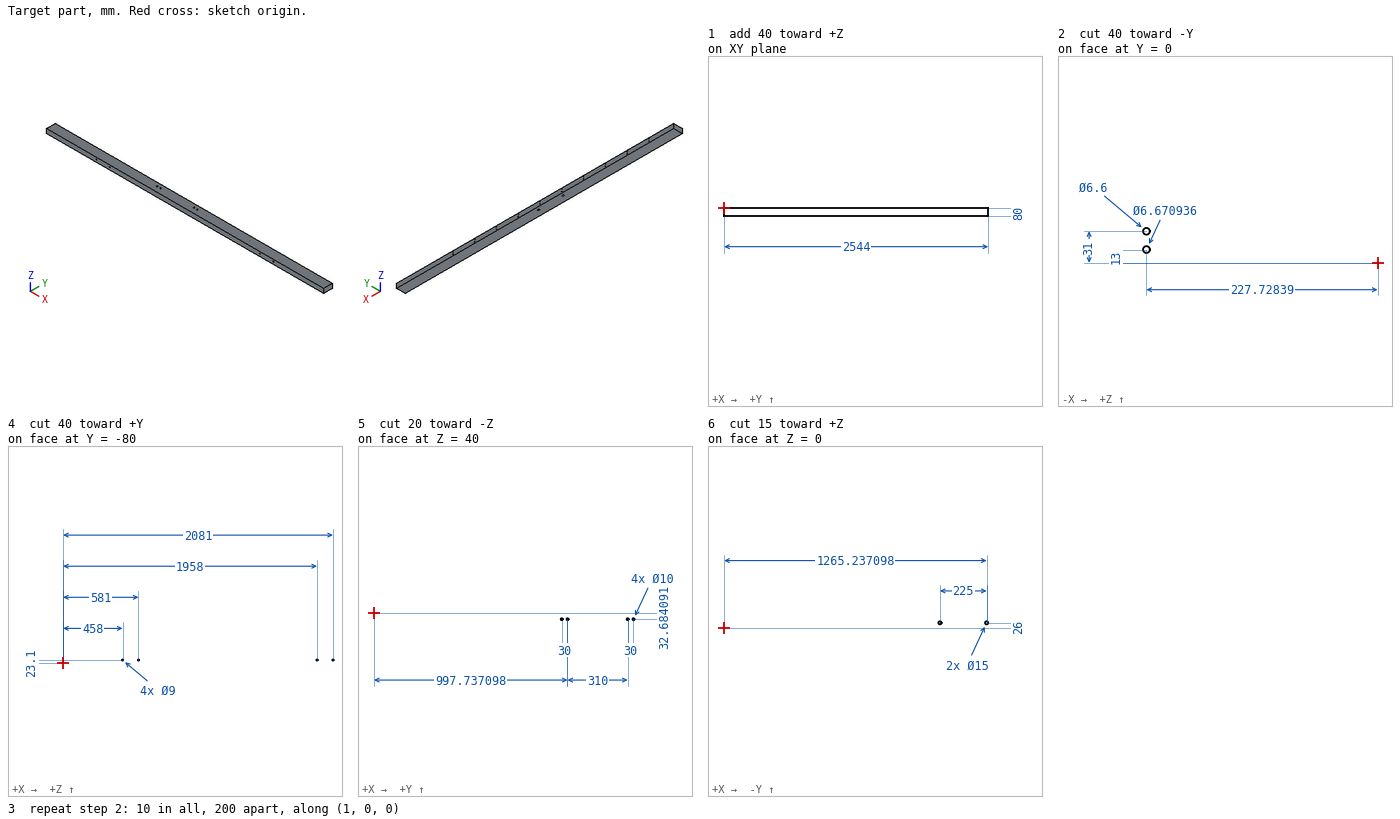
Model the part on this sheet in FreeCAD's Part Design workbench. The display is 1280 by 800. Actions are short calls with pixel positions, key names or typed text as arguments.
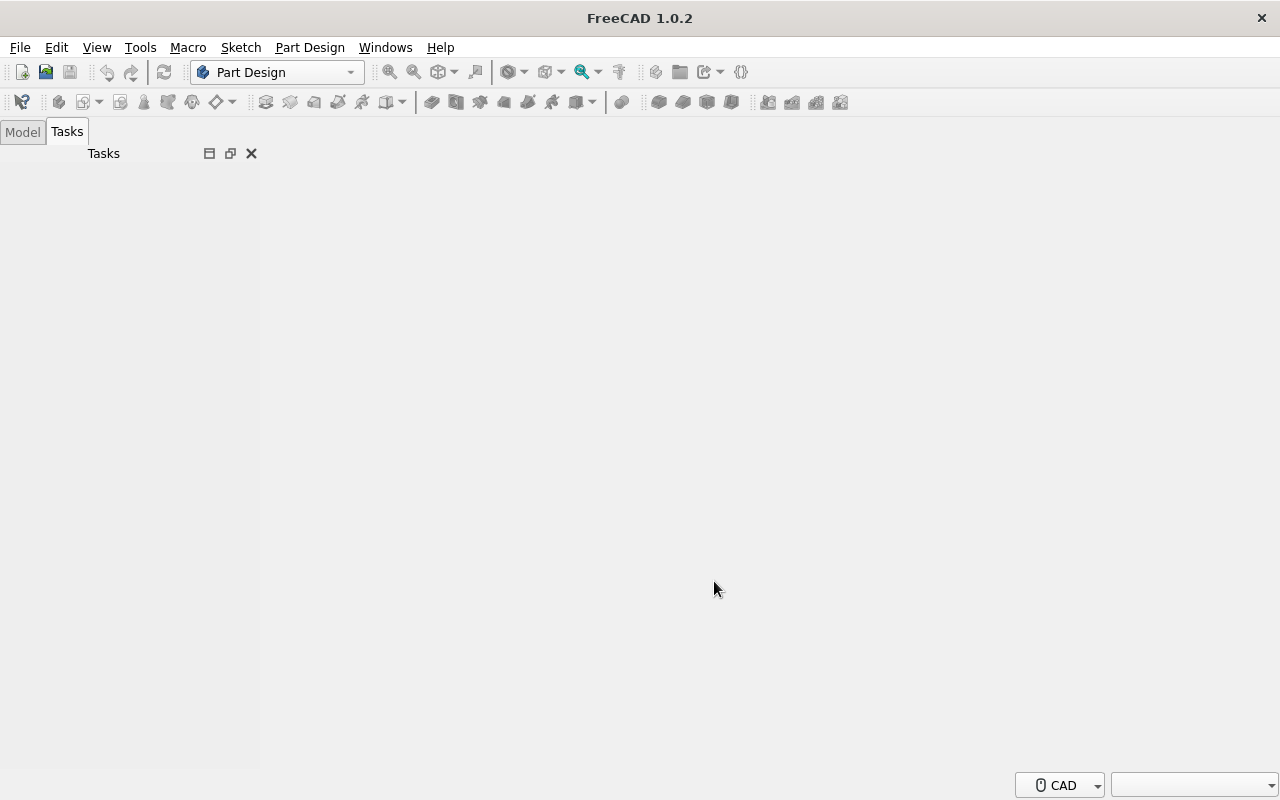
key(ctrl+n)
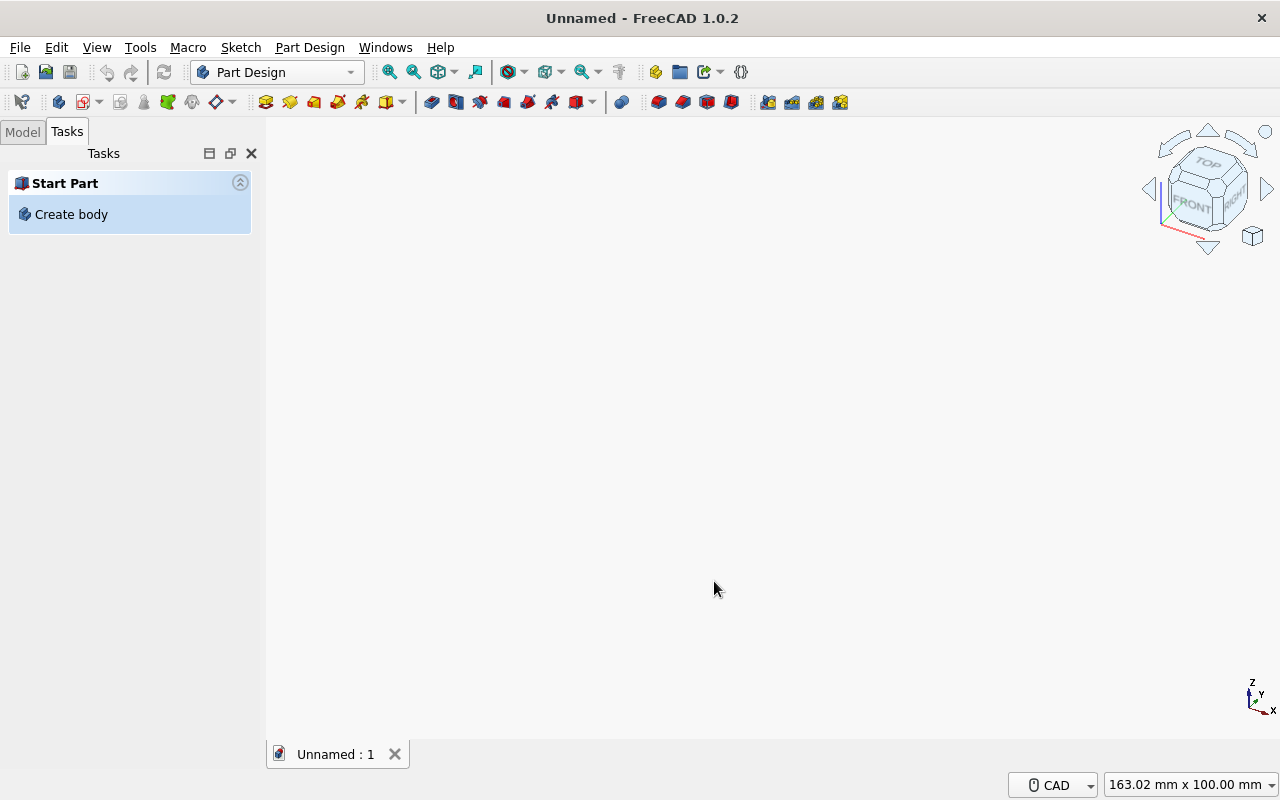
click(84, 102)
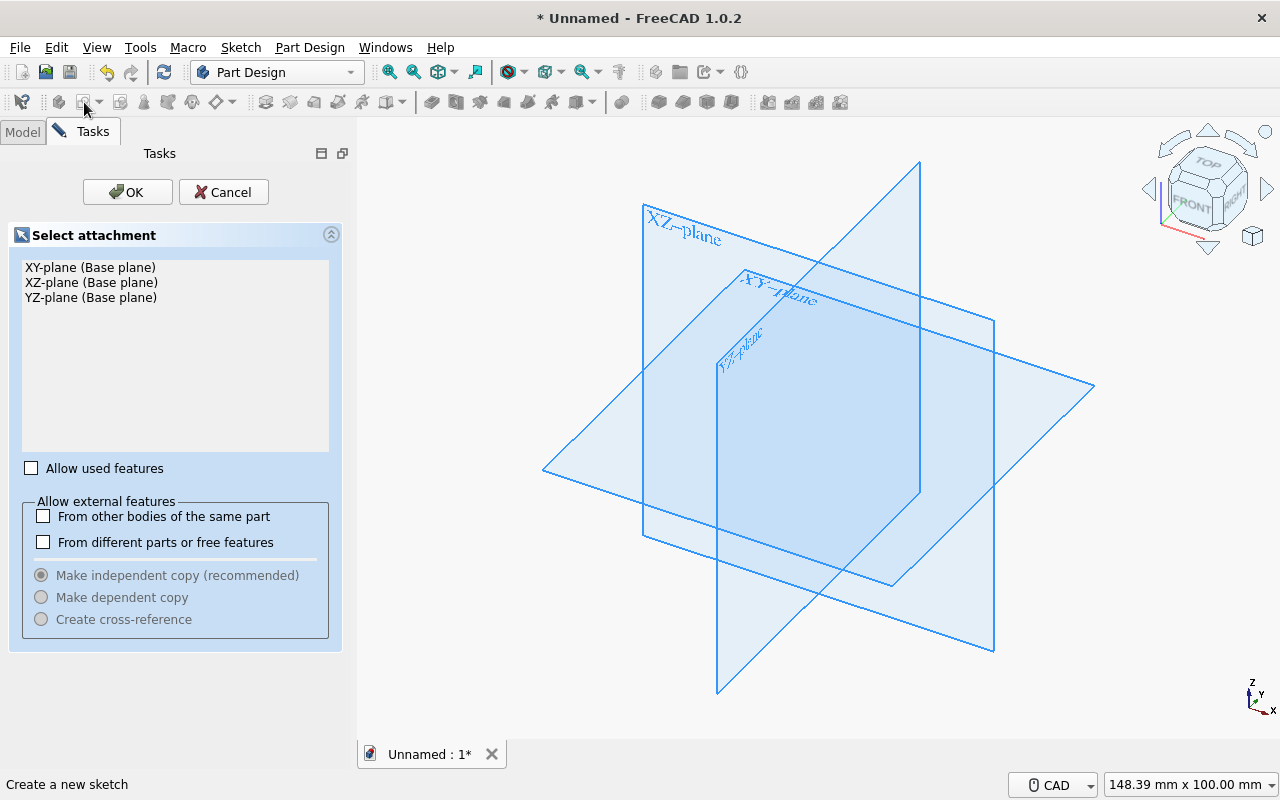
click(82, 268)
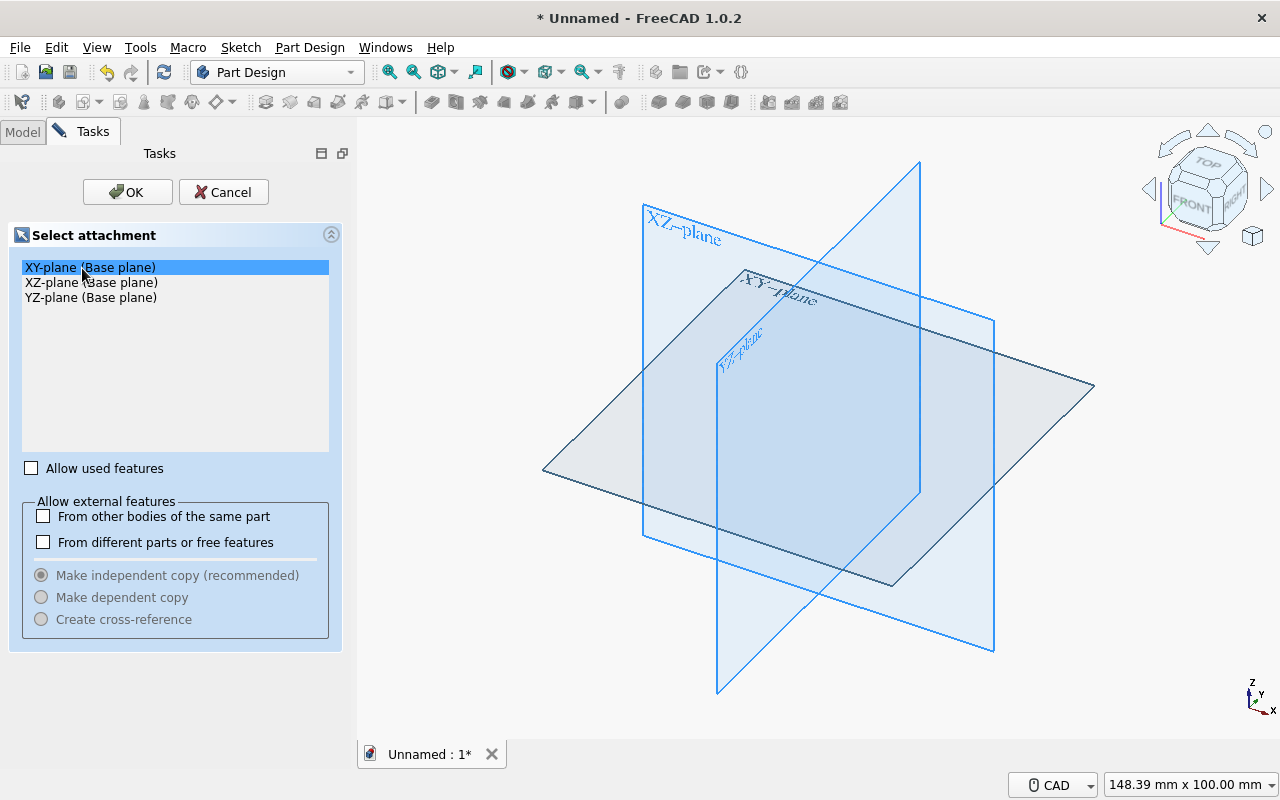
click(128, 192)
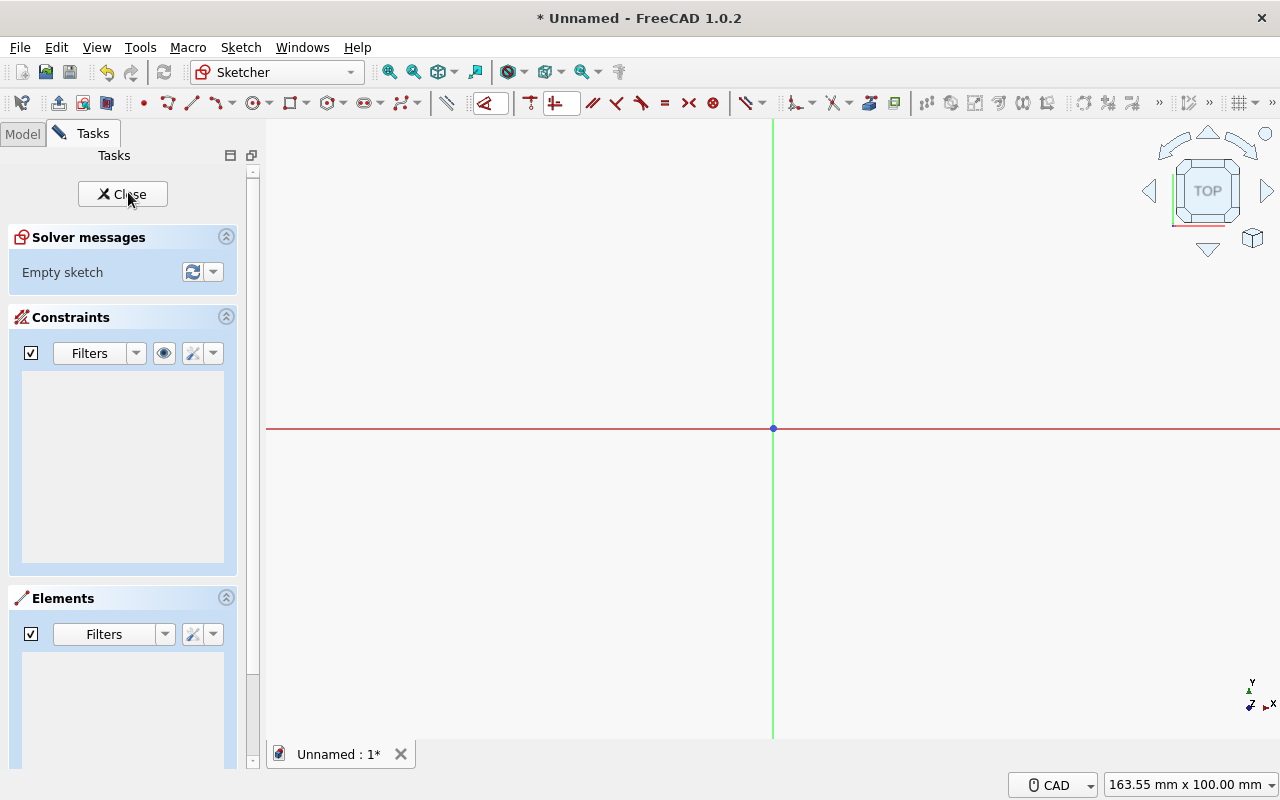
scroll(366, 418, down, 16)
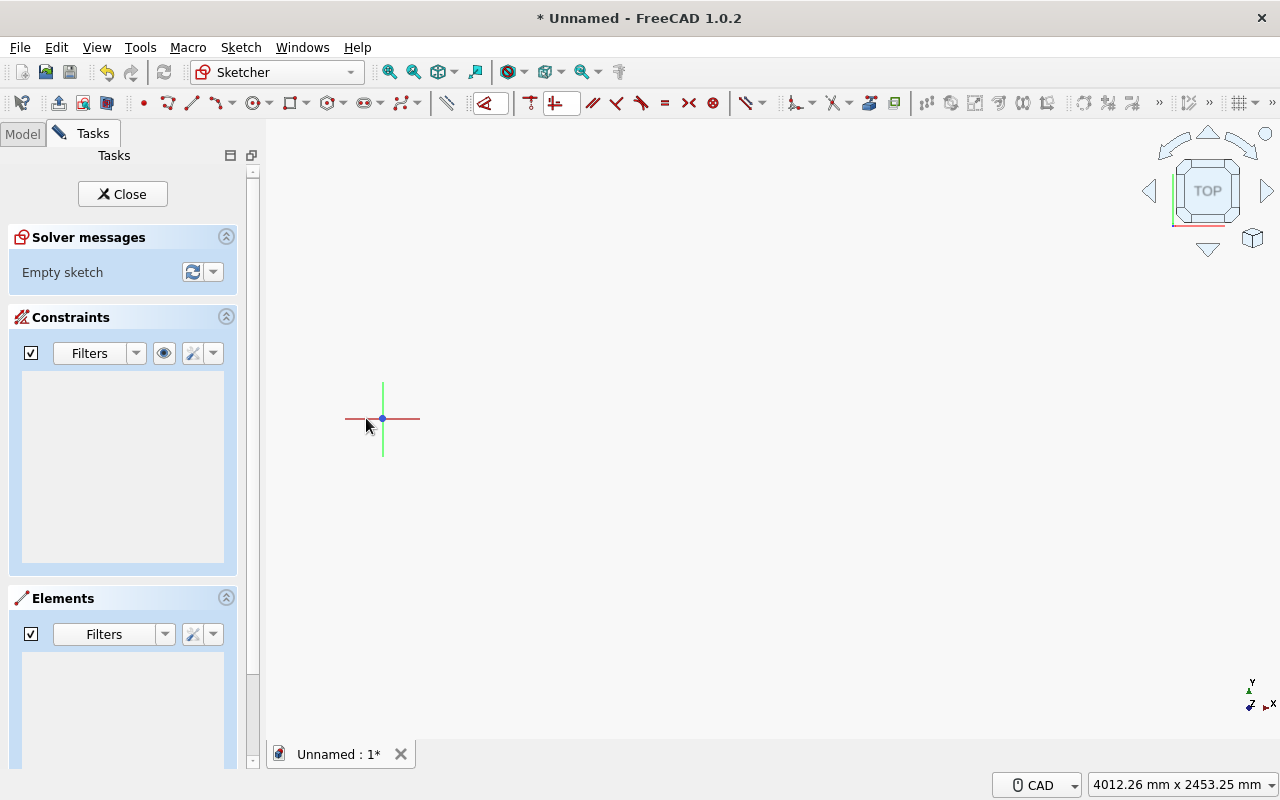
key(g)
key(r)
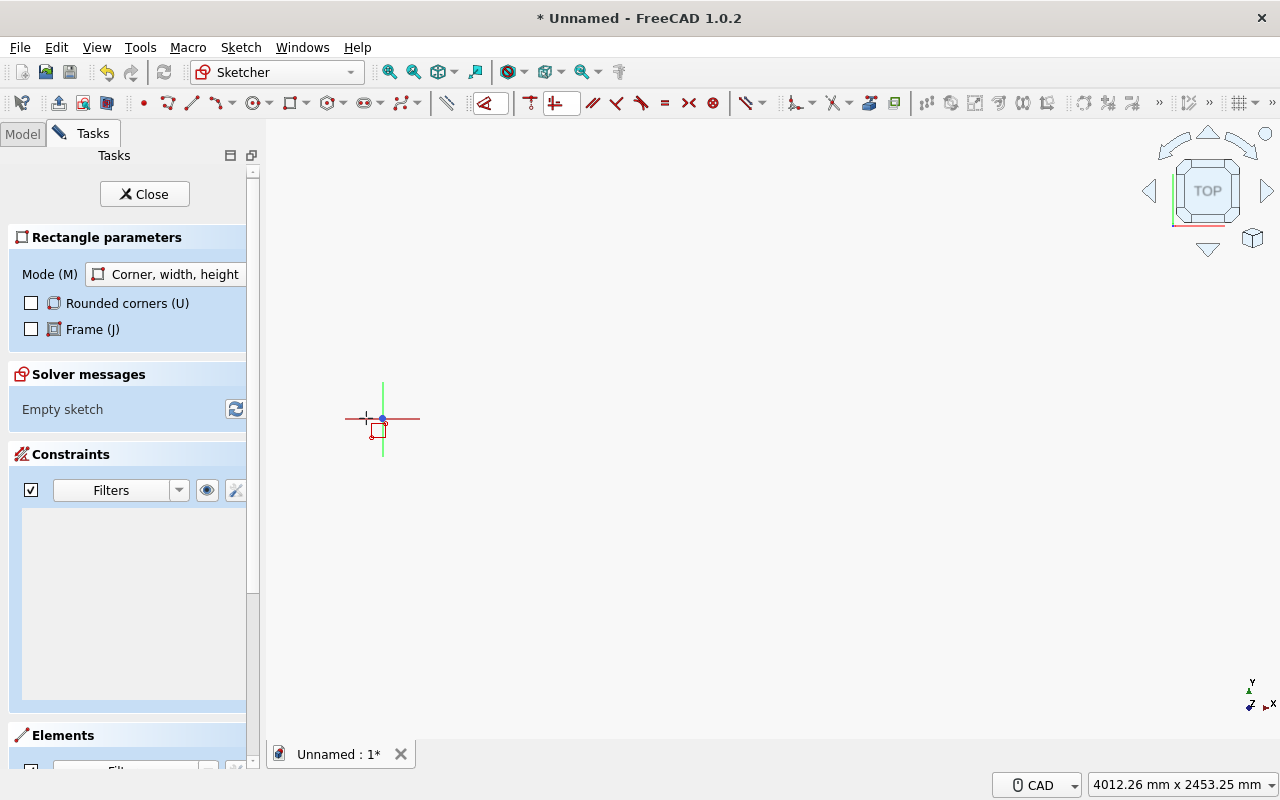
click(383, 419)
move(1026, 439)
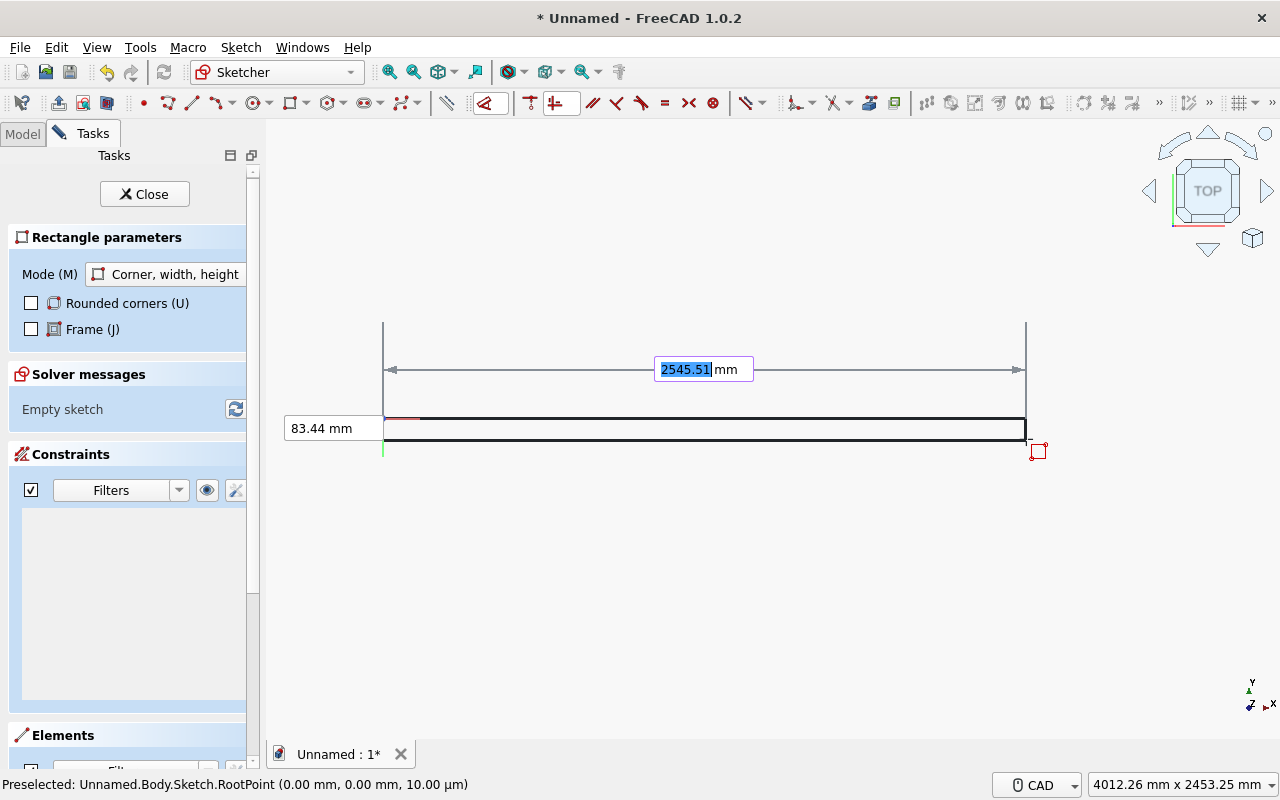
text(2544)
key(Tab)
text(80)
key(Return)
key(Escape)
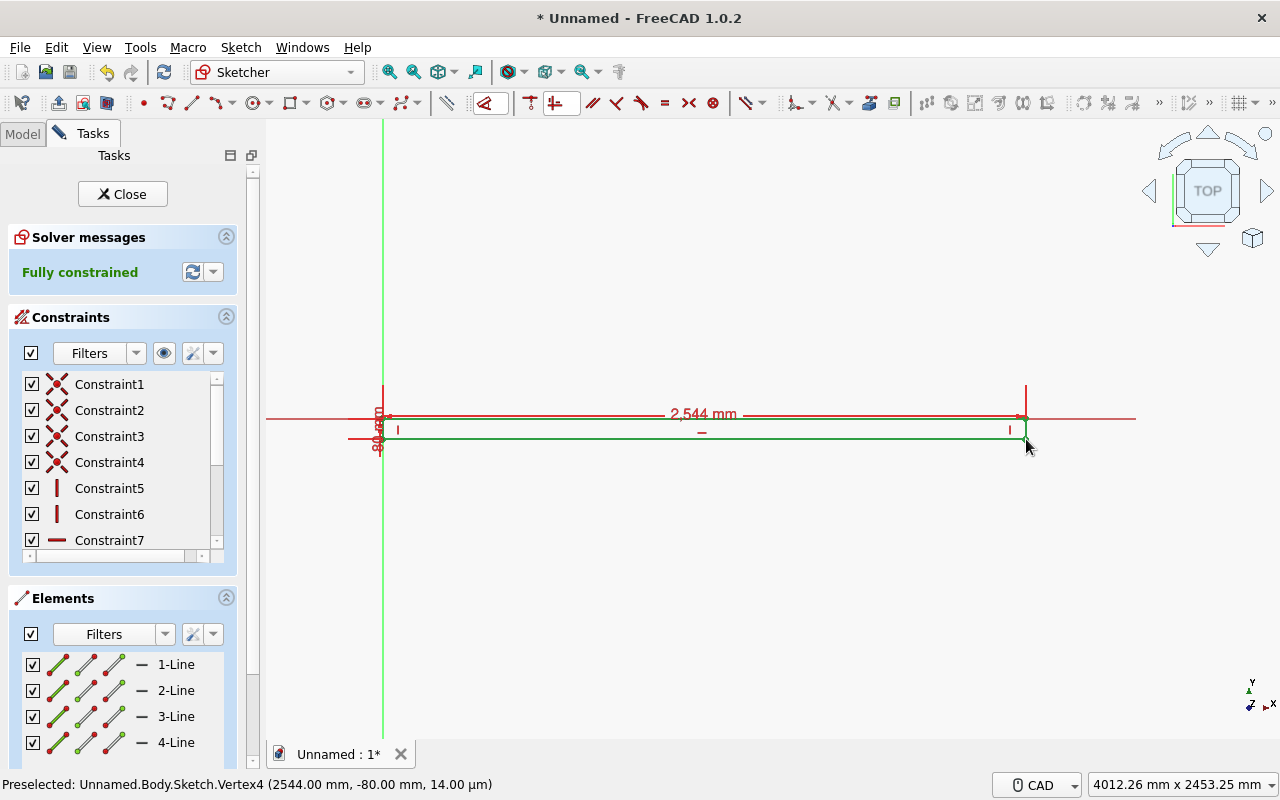
click(123, 194)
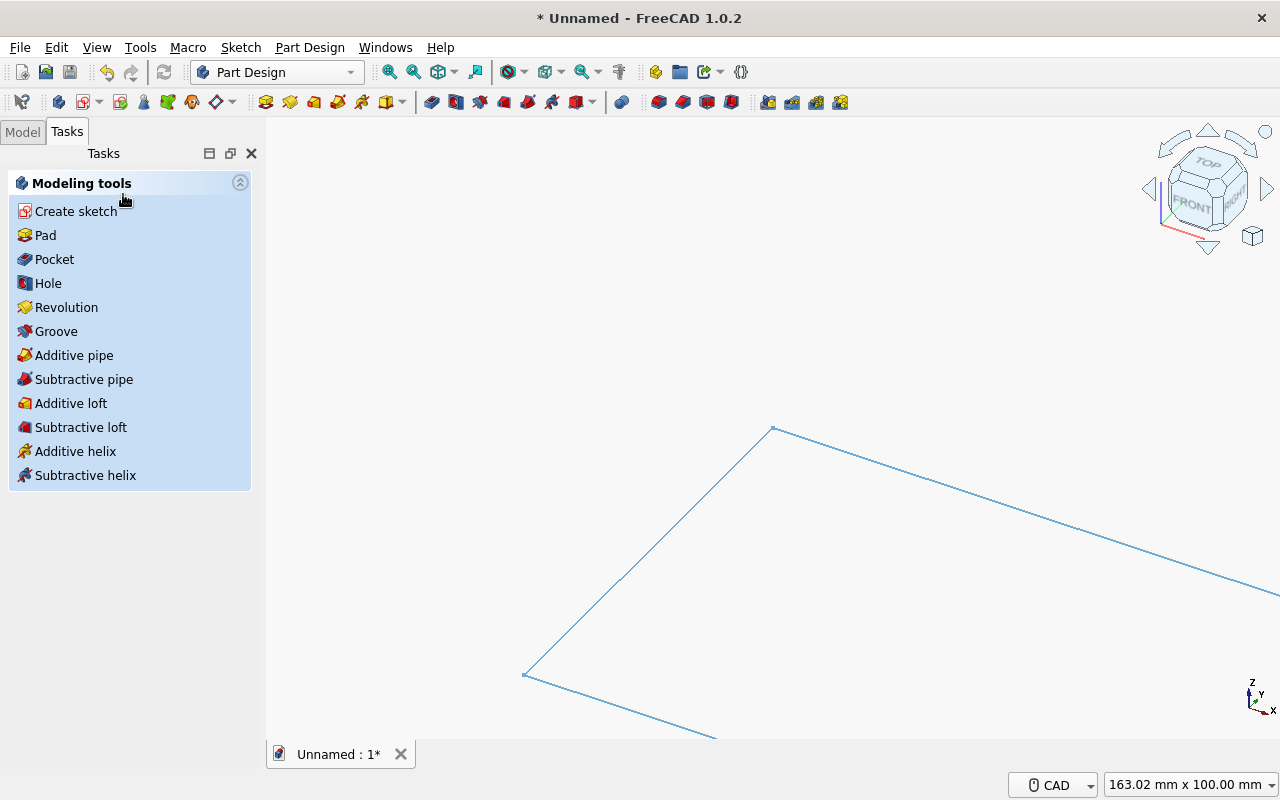
click(266, 102)